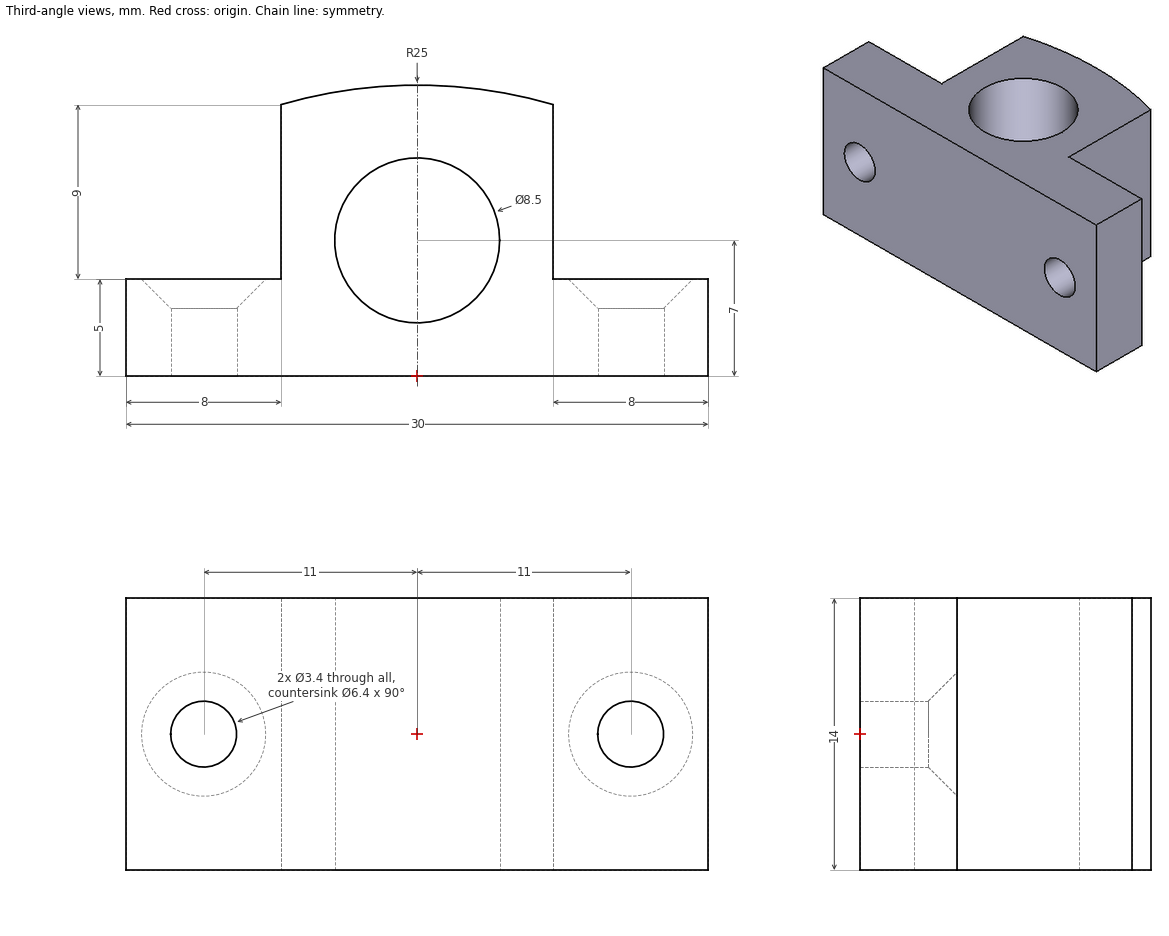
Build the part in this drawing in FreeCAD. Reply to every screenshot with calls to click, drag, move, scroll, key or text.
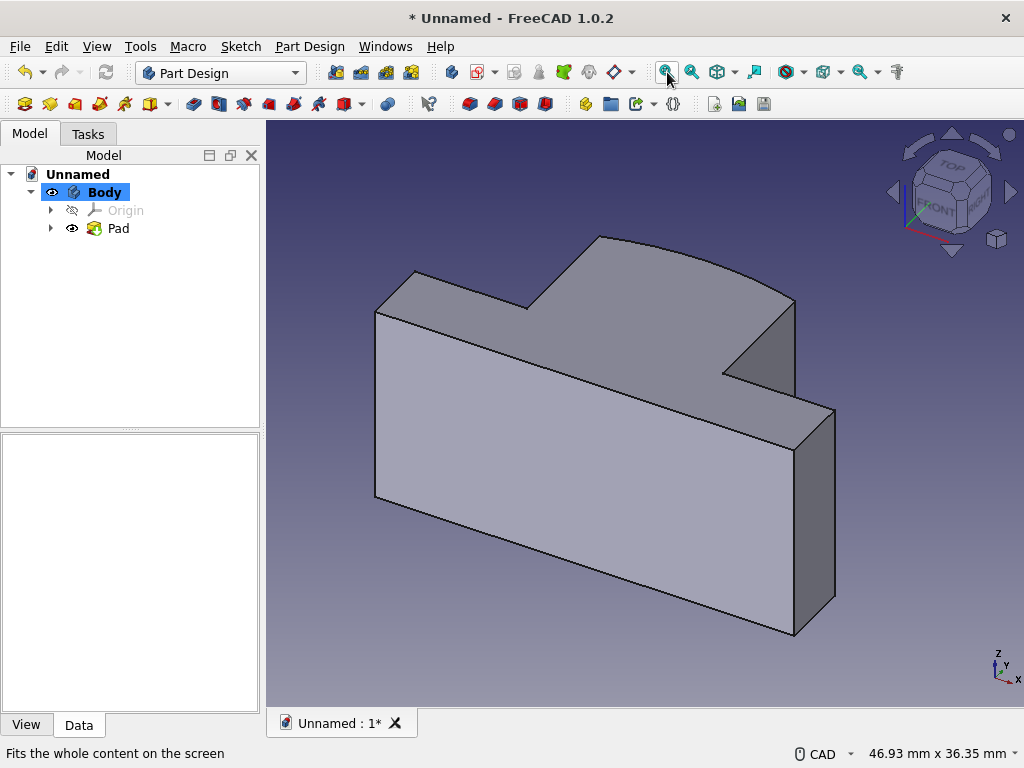
key(4)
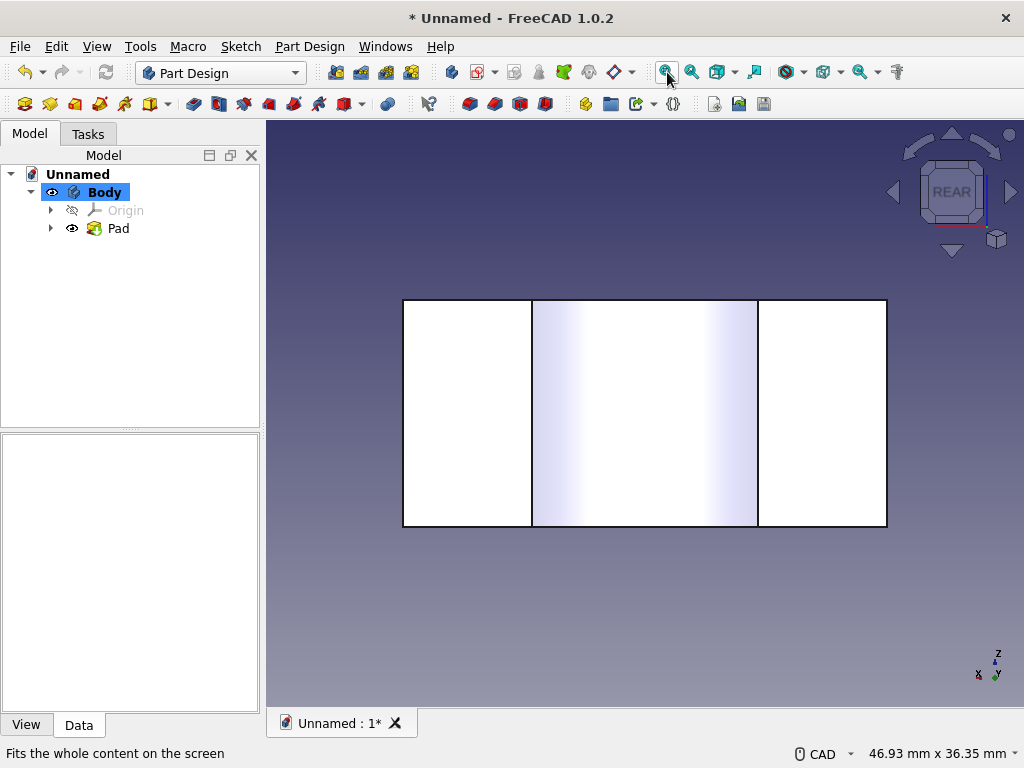
click(823, 380)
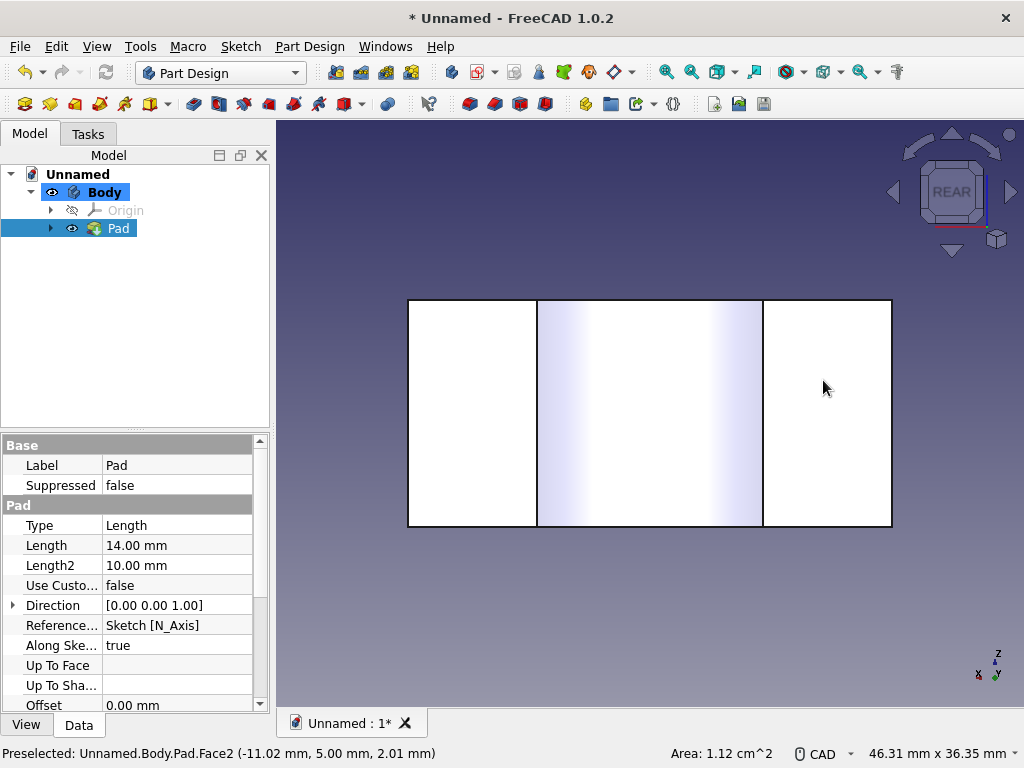
click(476, 72)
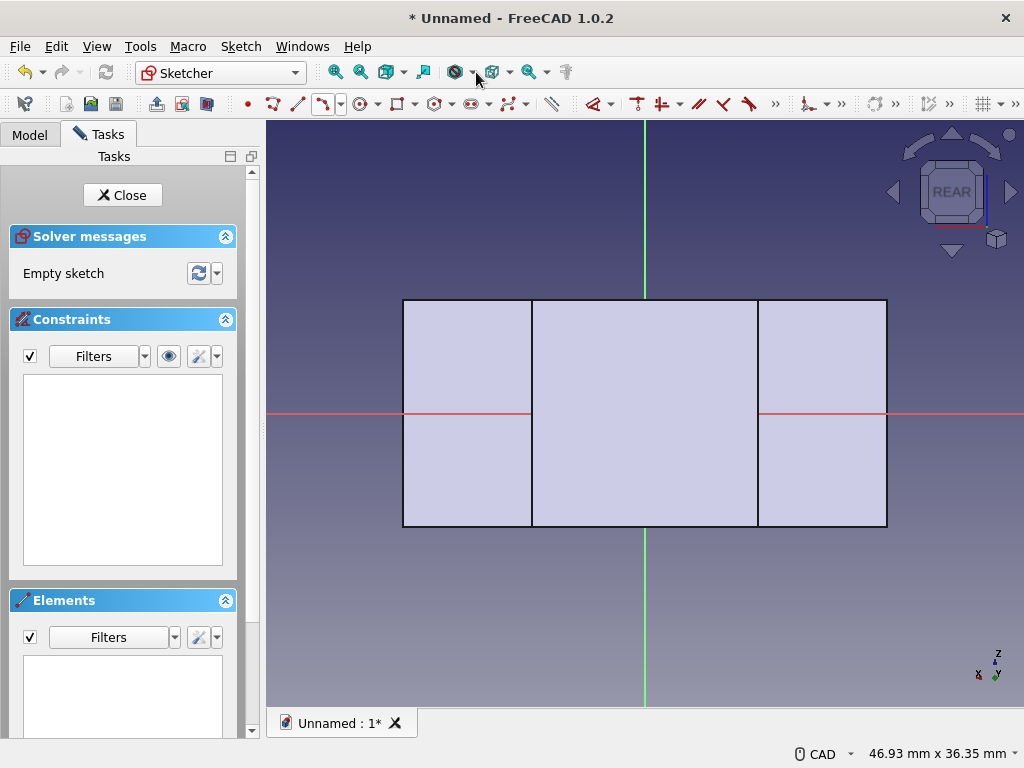
click(207, 104)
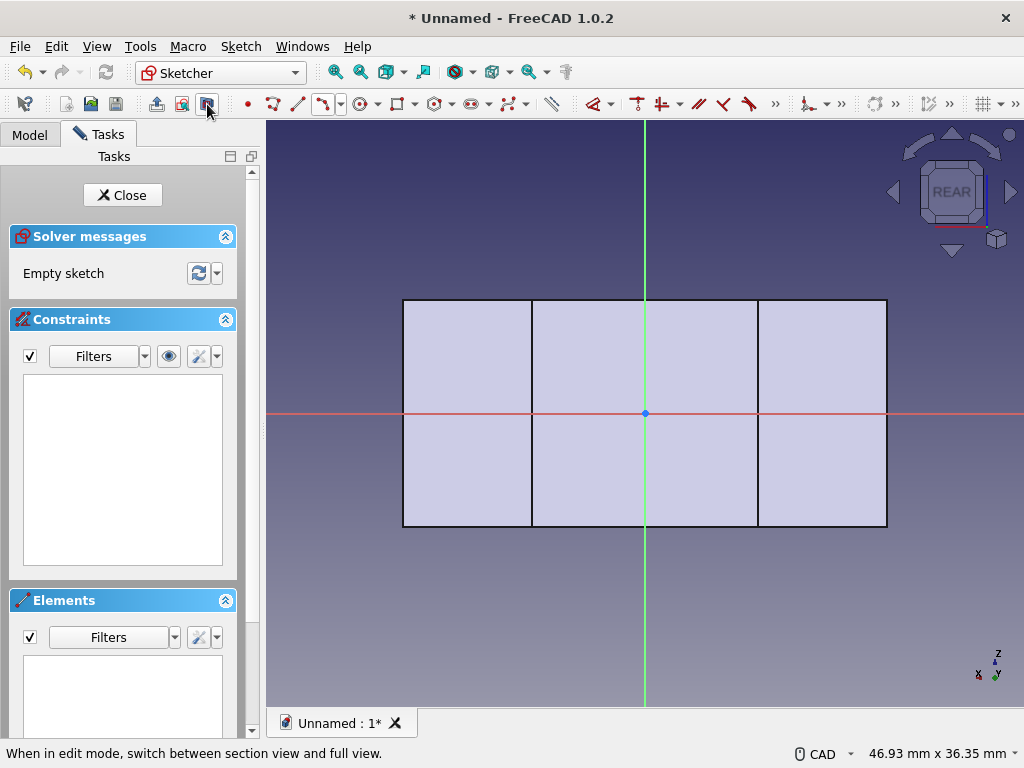
scroll(294, 414, down, 1)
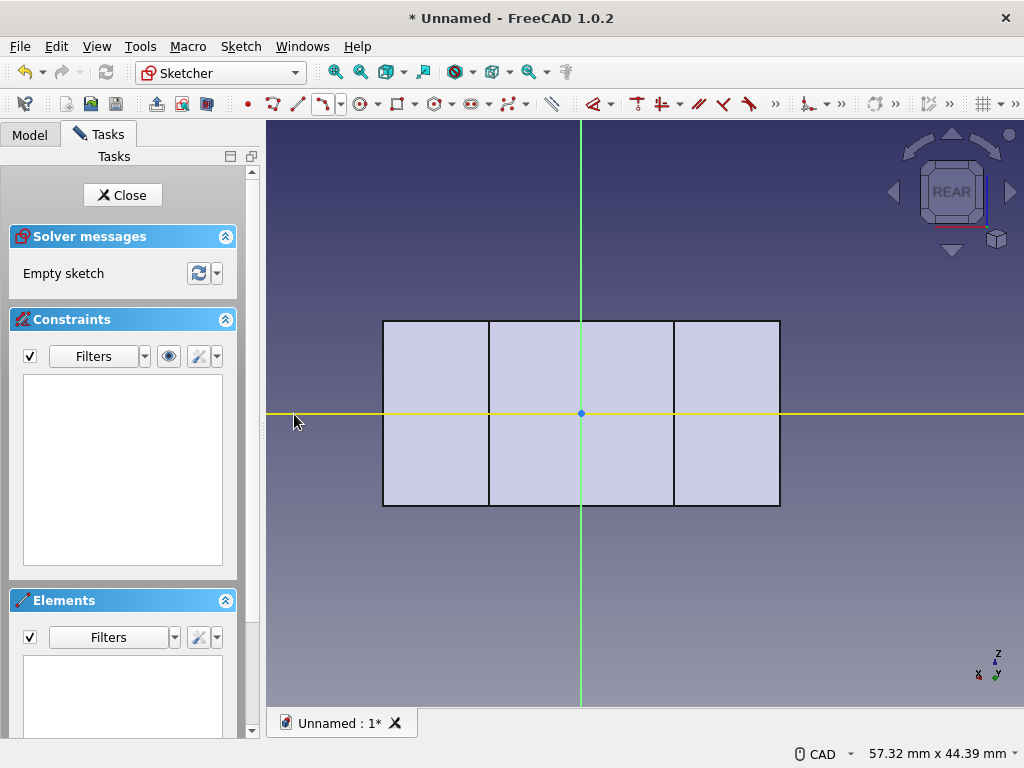
click(360, 104)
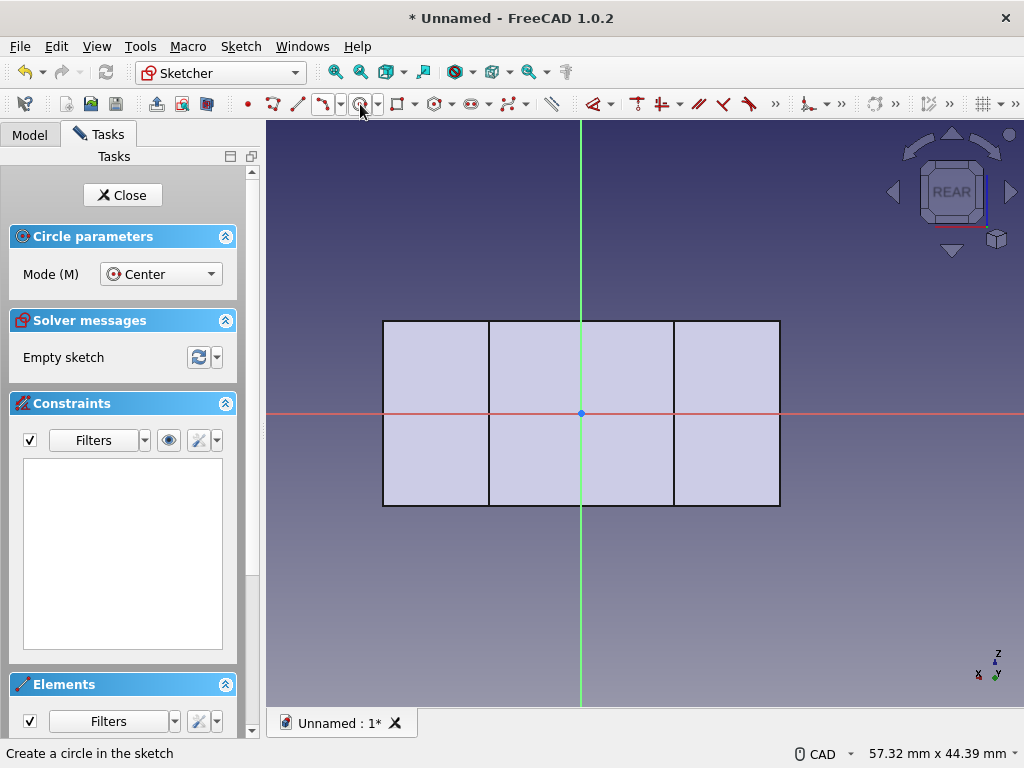
click(727, 414)
move(743, 398)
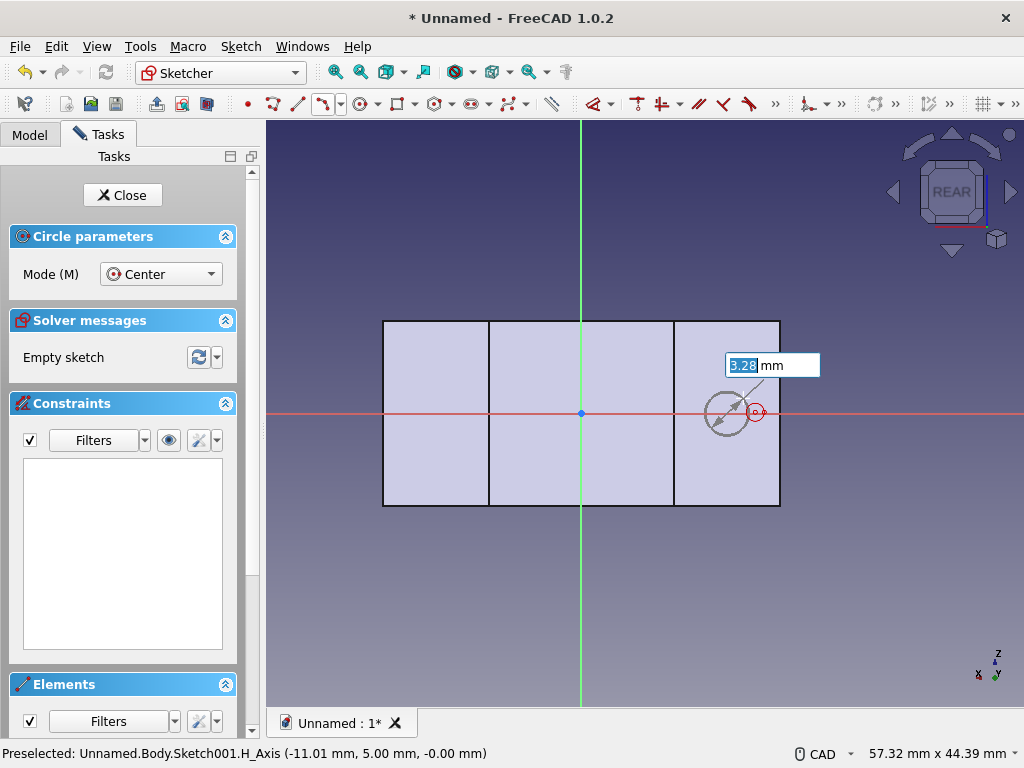
text(3.4)
key(Return)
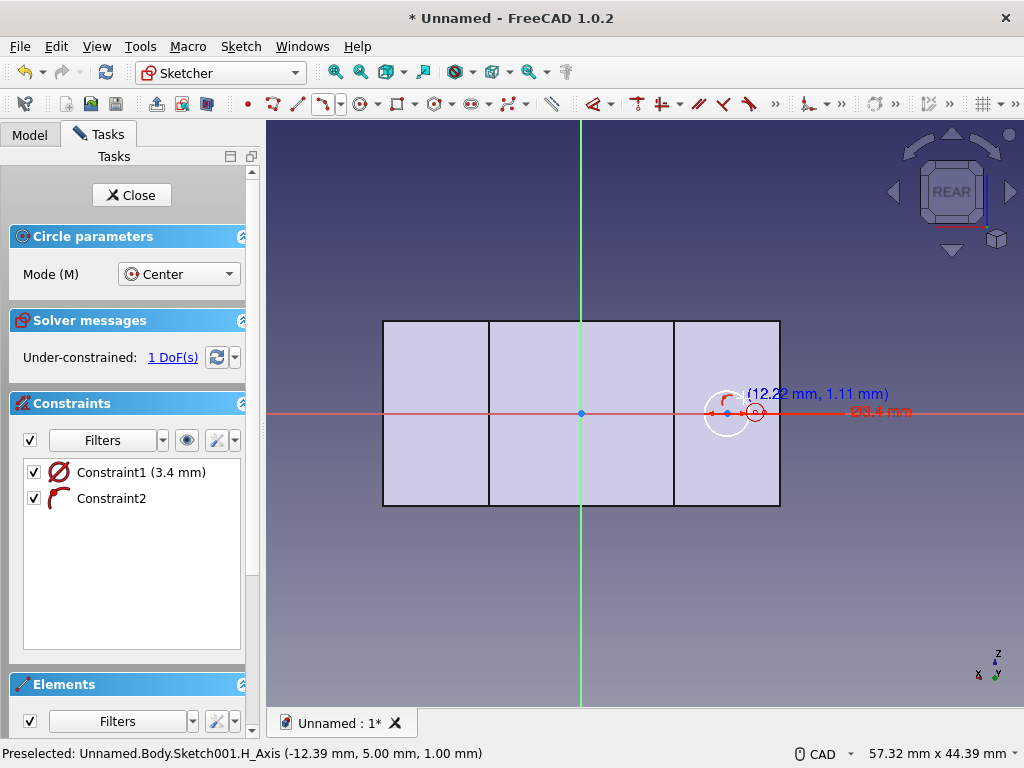
click(436, 414)
move(452, 398)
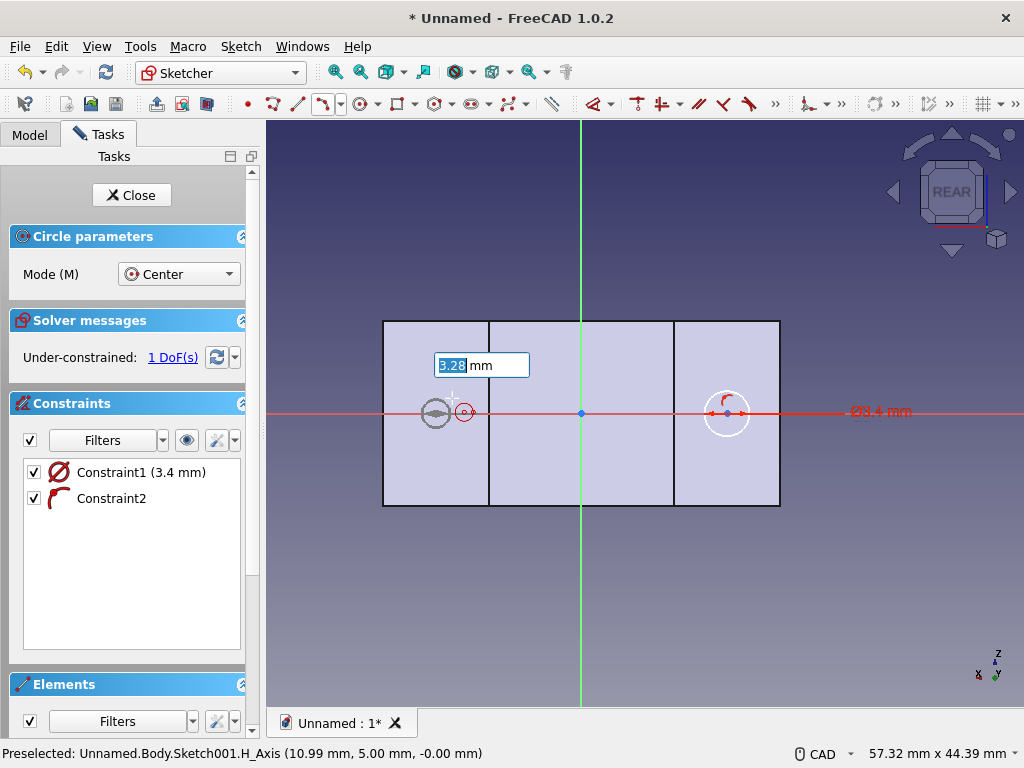
text(3.4)
key(Return)
key(Escape)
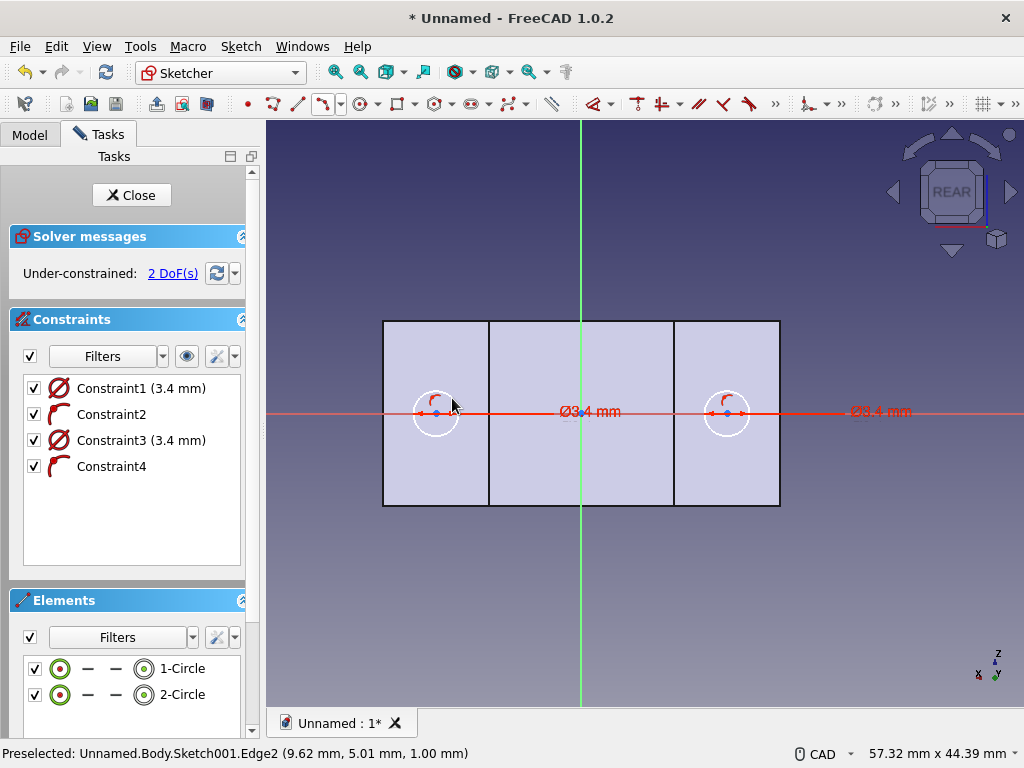
click(592, 104)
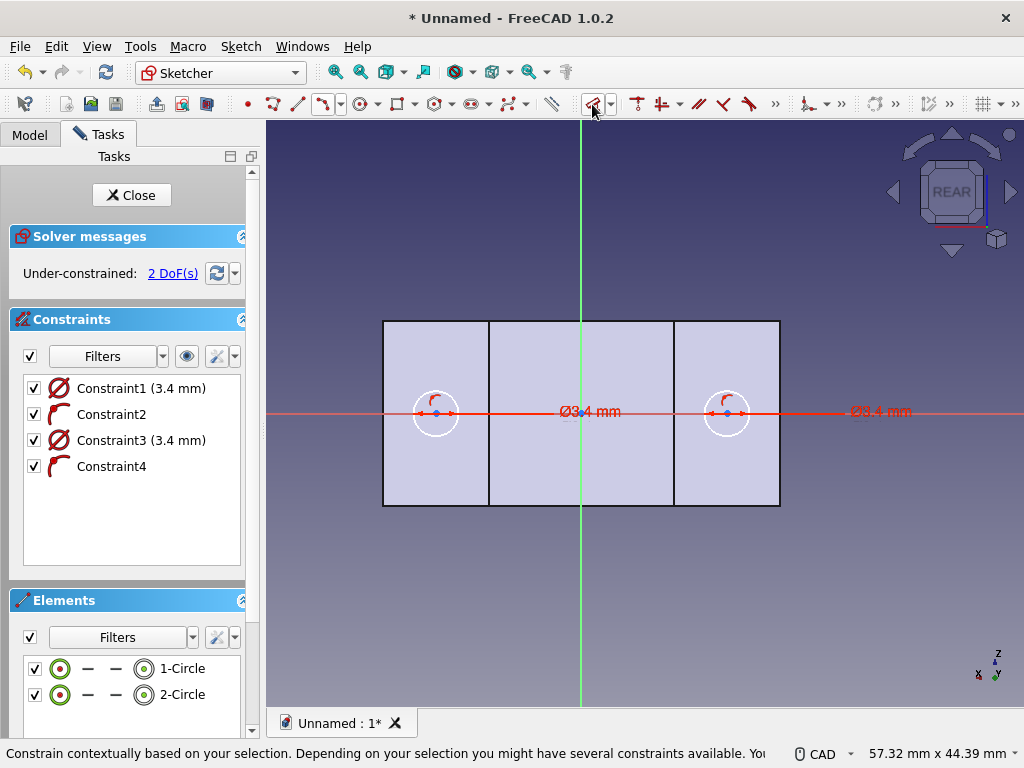
click(727, 414)
click(654, 448)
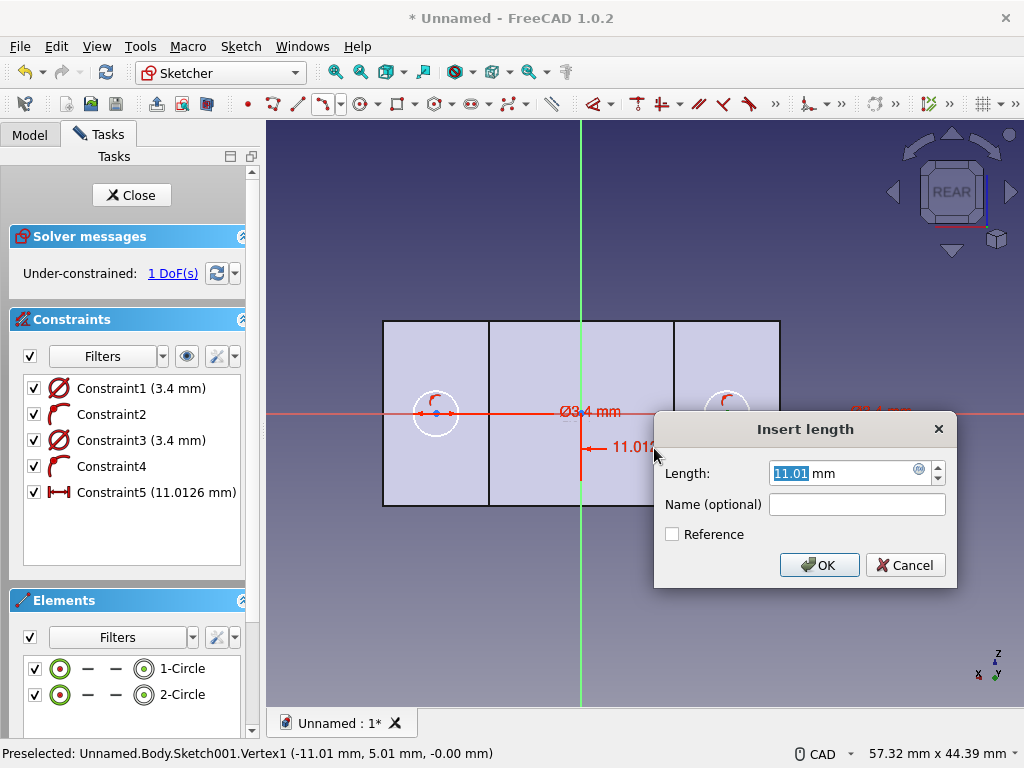
text(11)
key(Return)